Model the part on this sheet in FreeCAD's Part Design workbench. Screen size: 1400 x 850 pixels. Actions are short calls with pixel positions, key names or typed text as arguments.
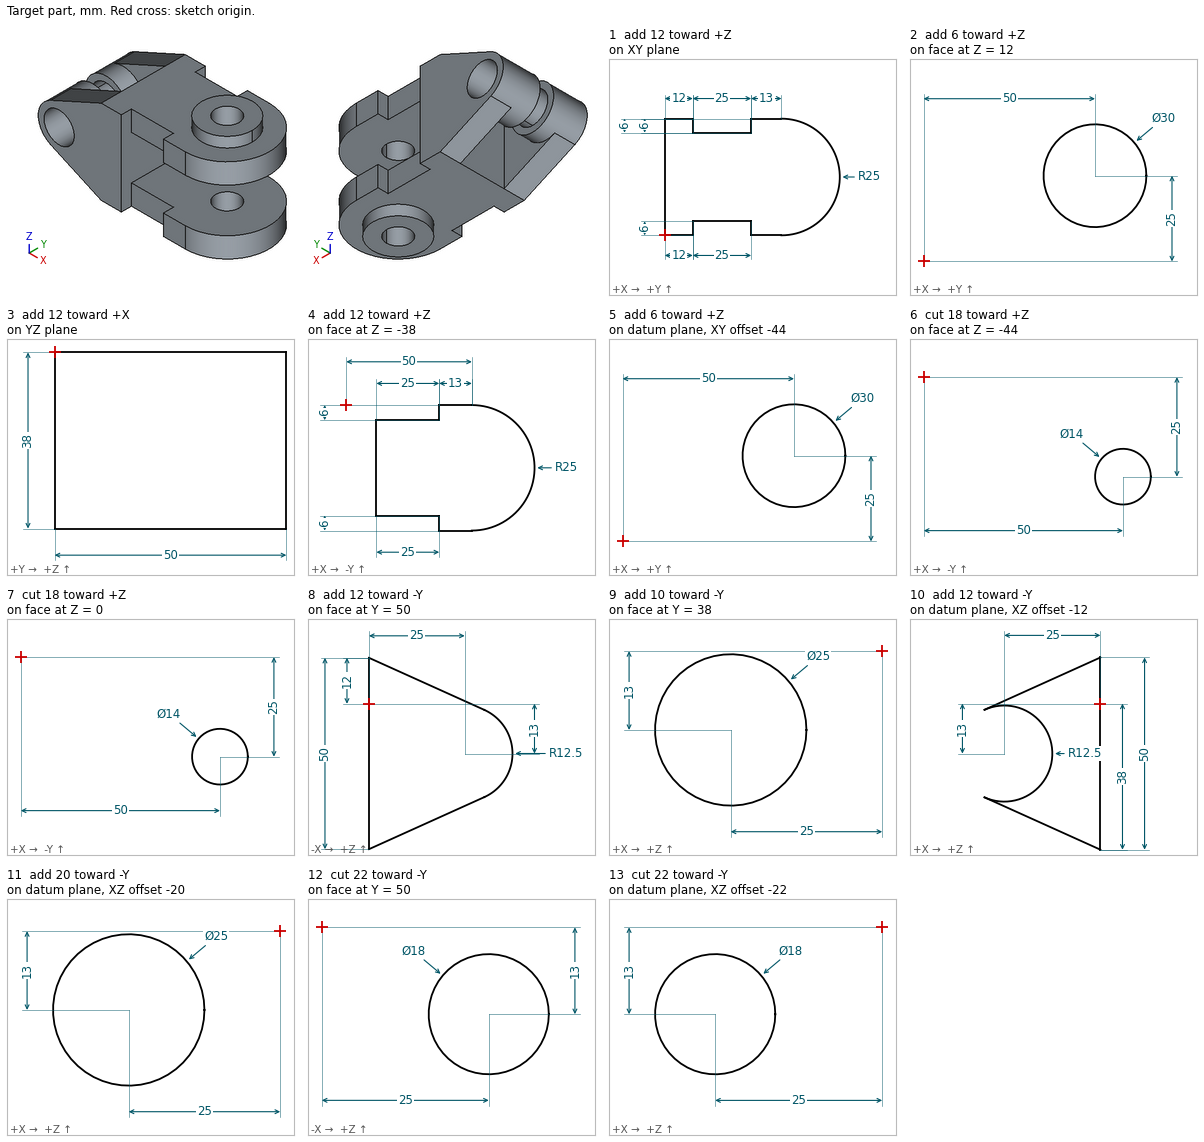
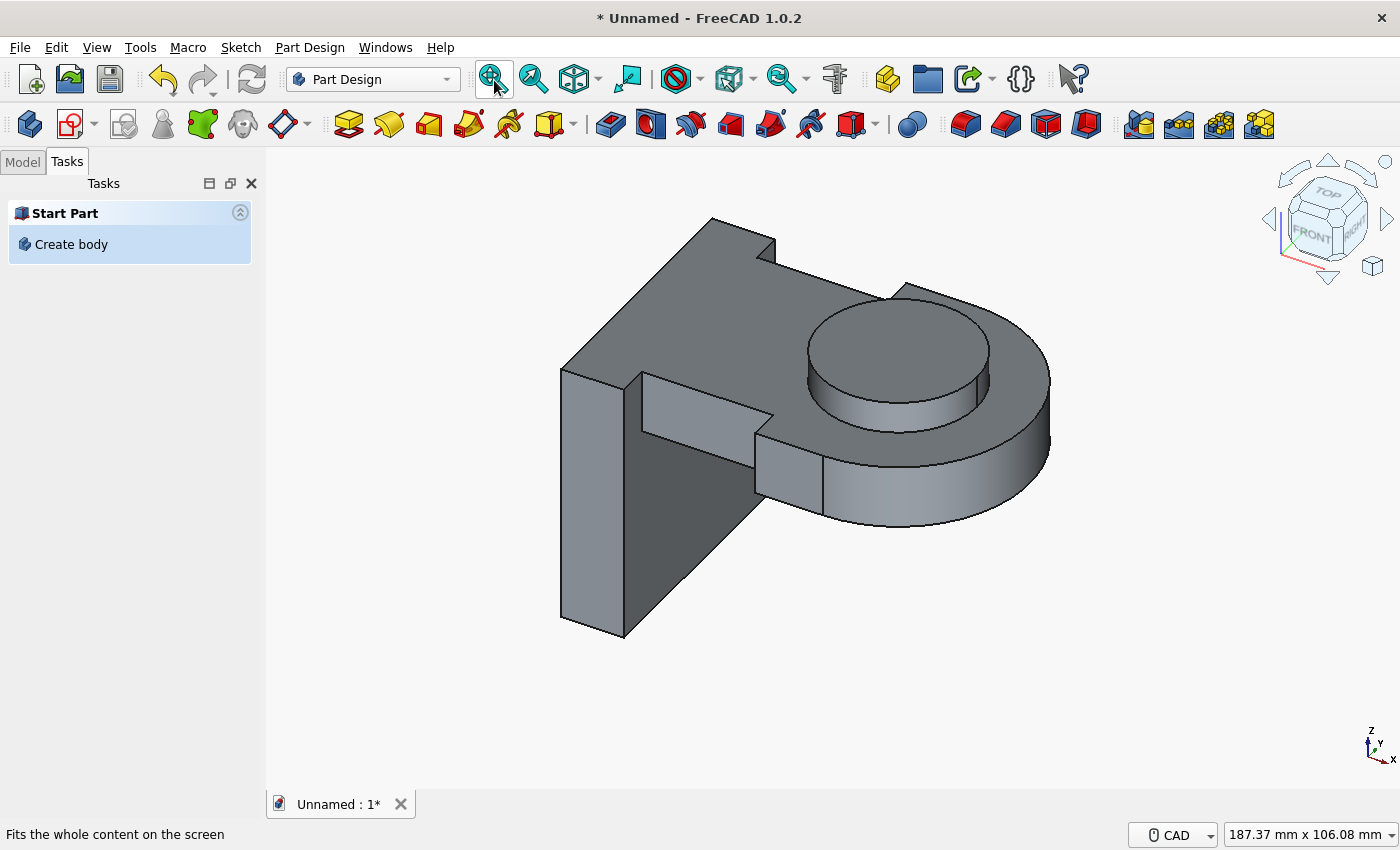
key(5)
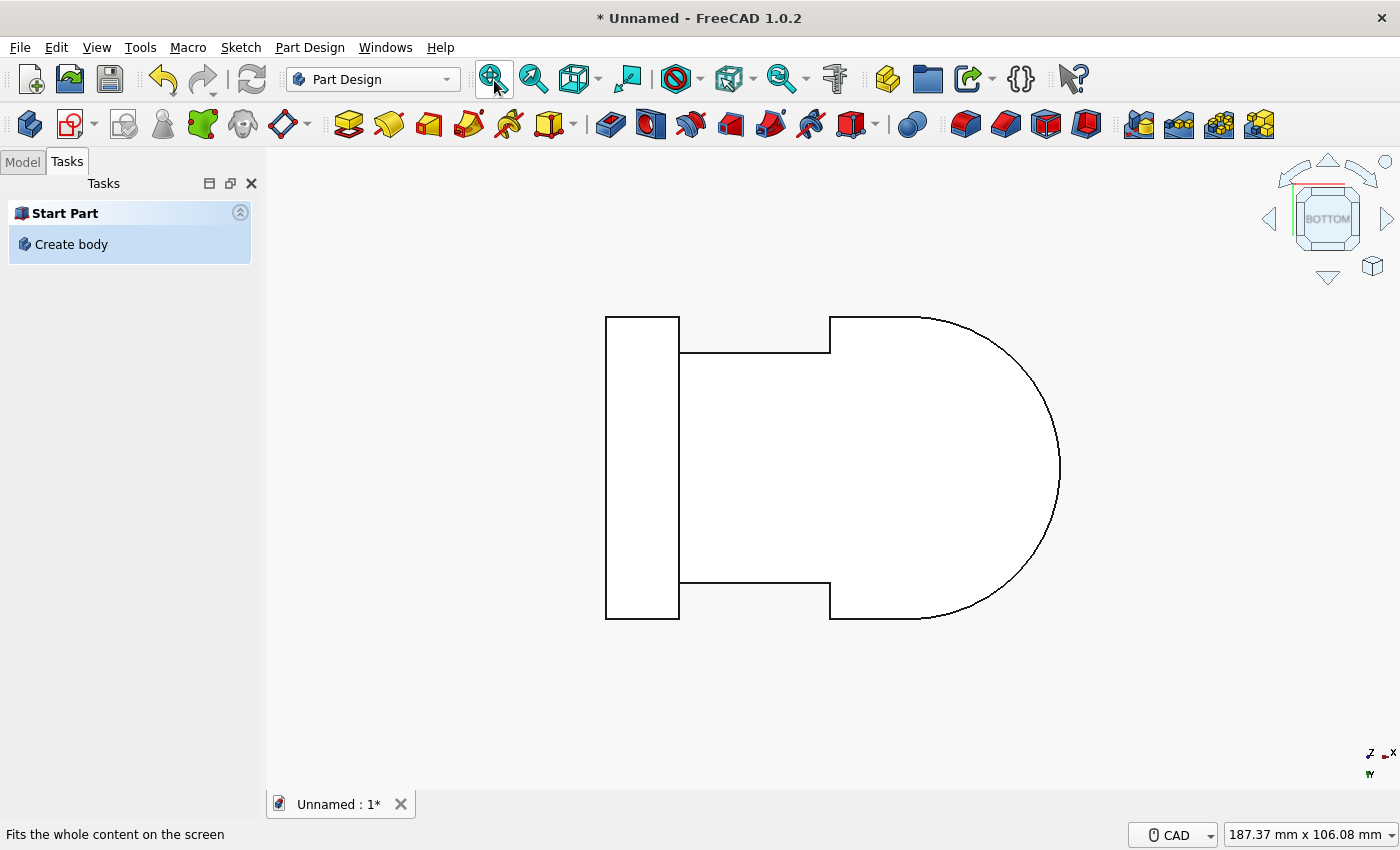
click(643, 553)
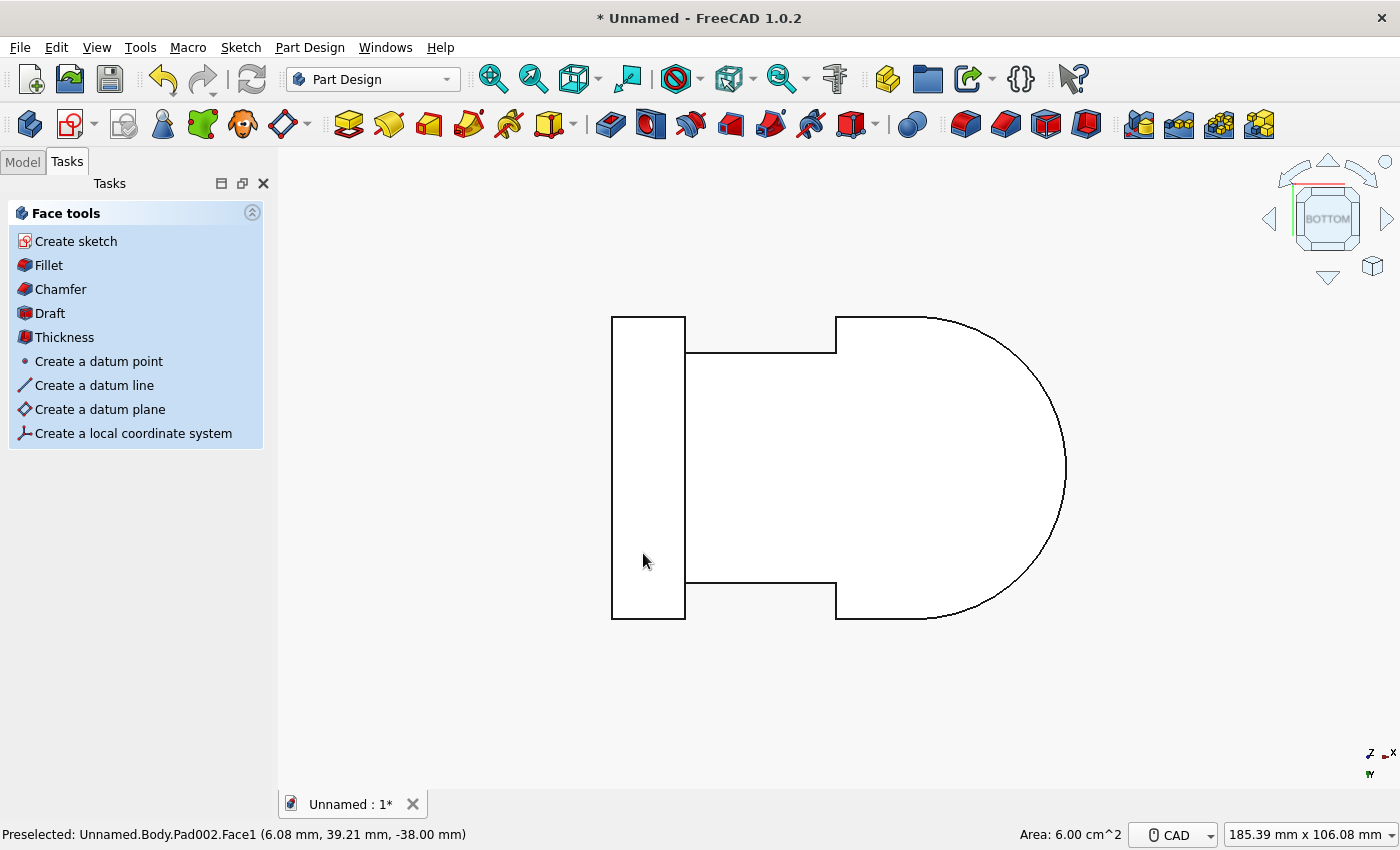
click(70, 124)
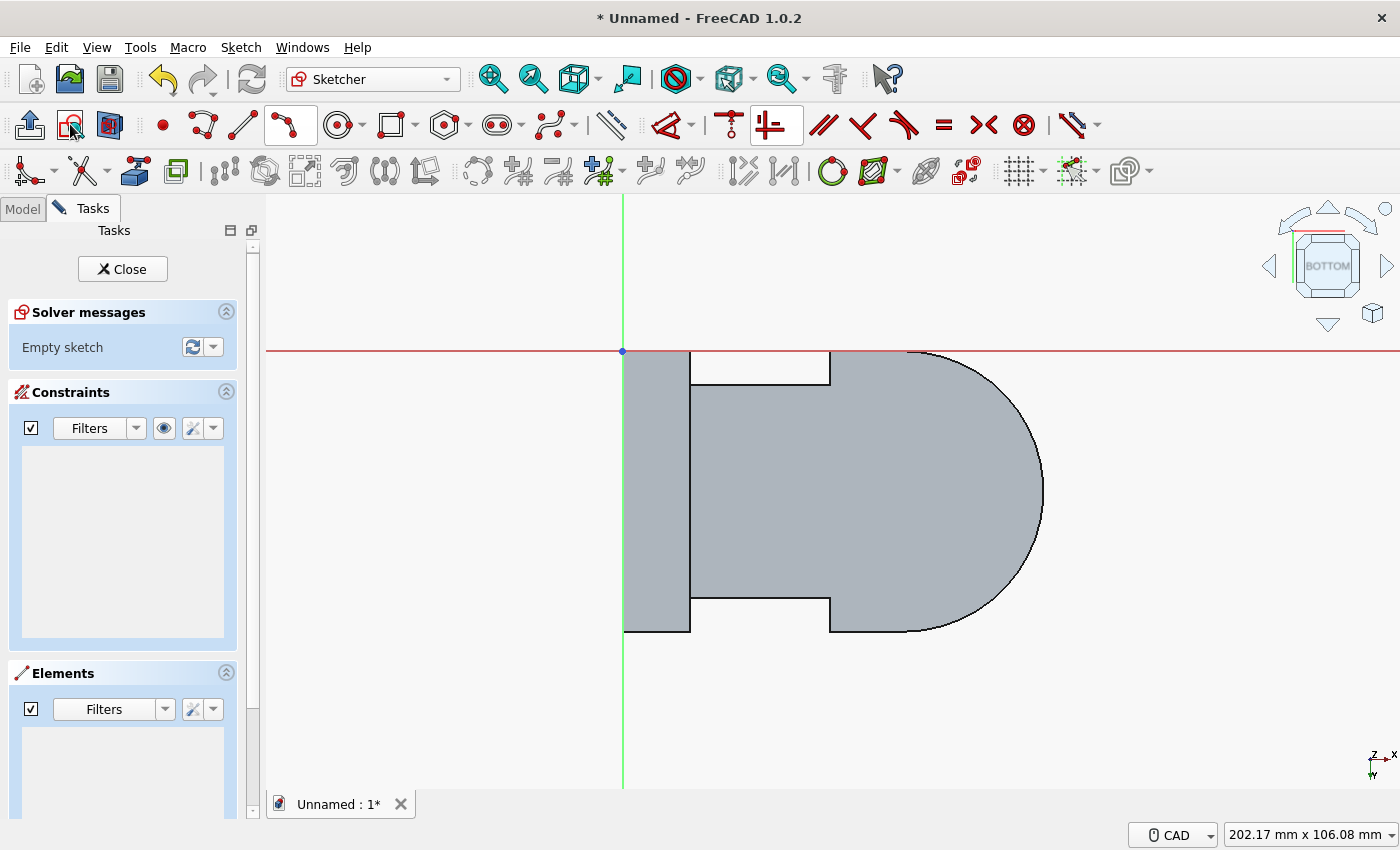
scroll(973, 491, up, 2)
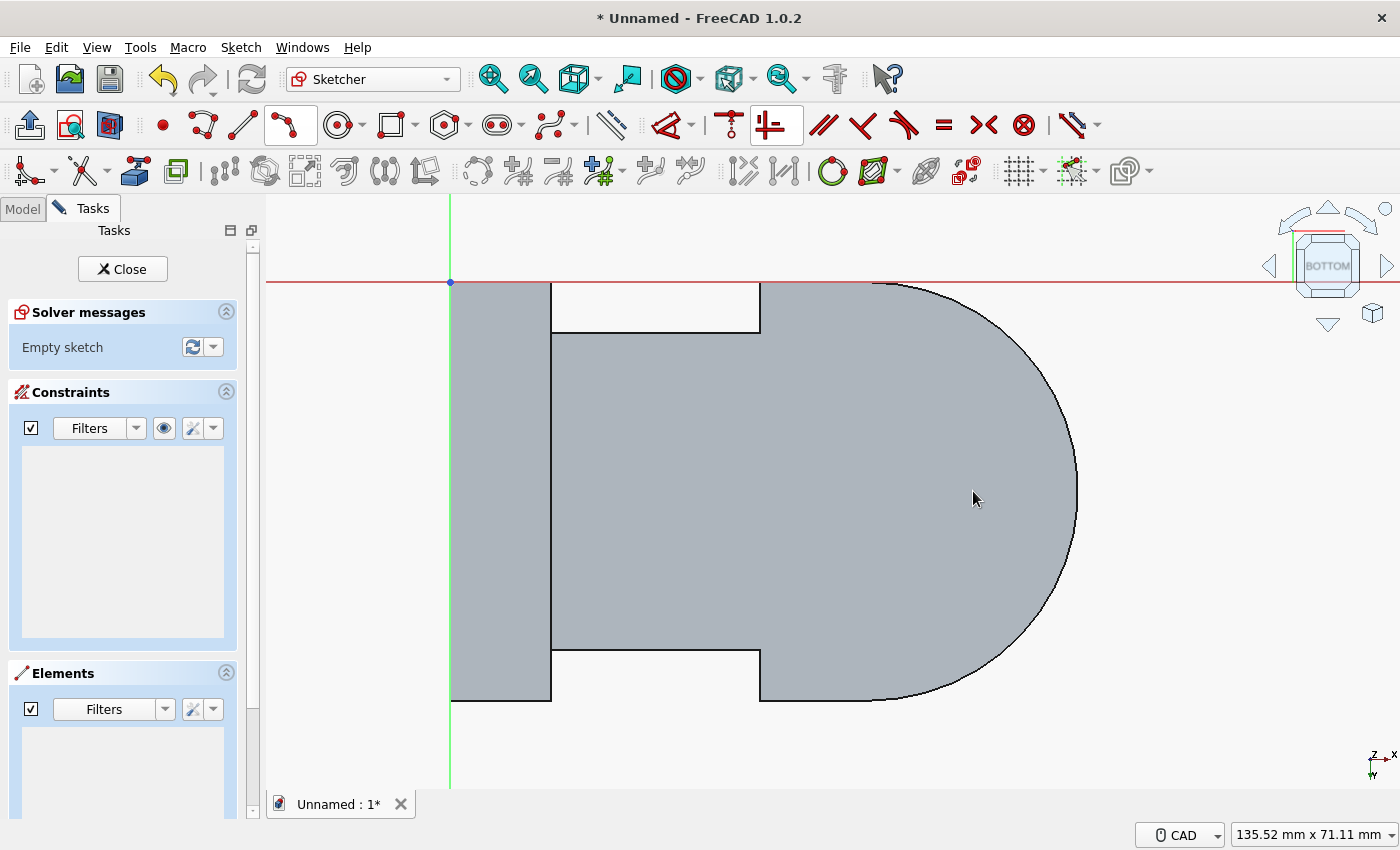
click(204, 126)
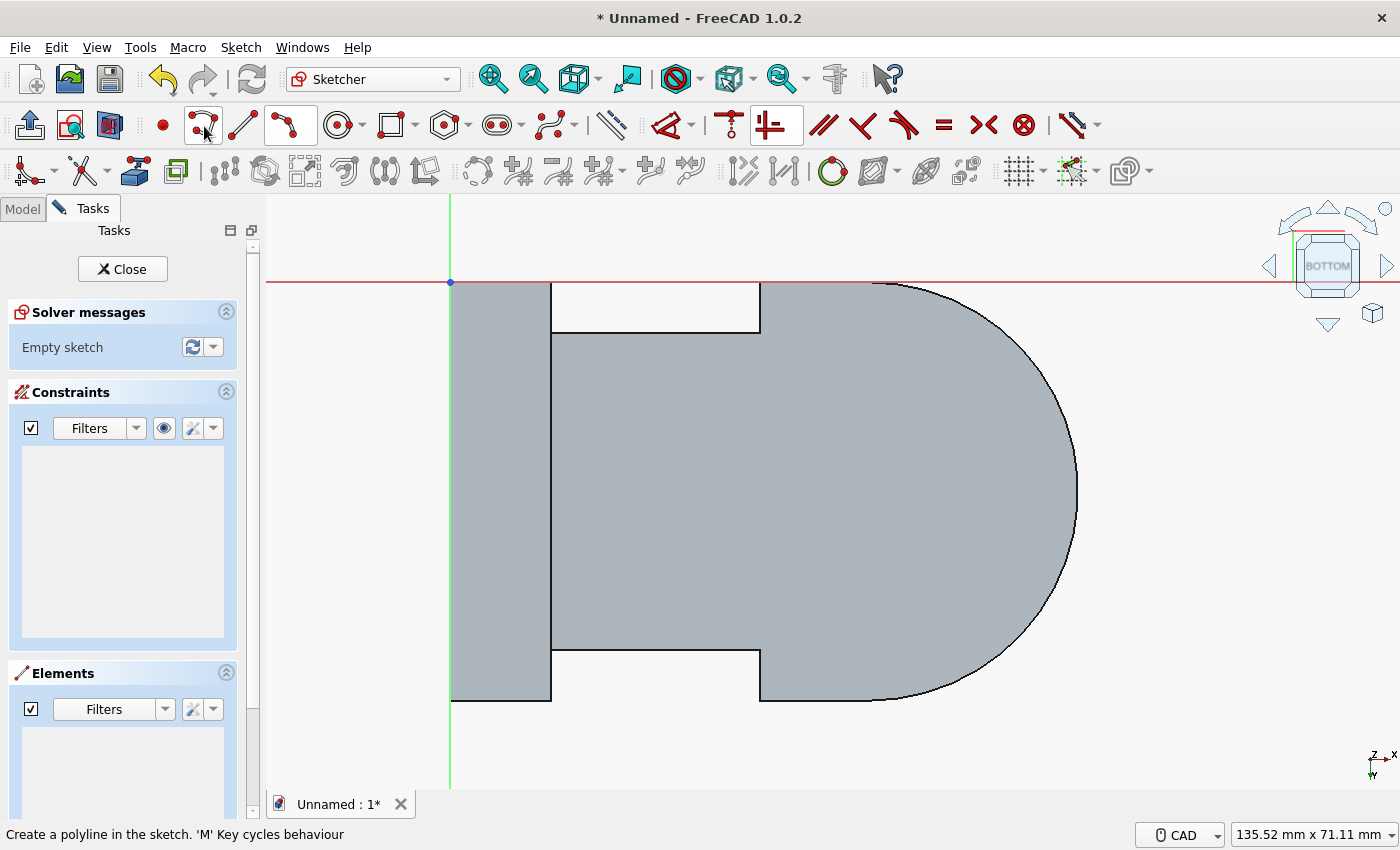
click(869, 282)
click(760, 291)
click(760, 333)
click(551, 333)
click(551, 650)
click(760, 650)
click(760, 701)
click(869, 701)
right_click(869, 701)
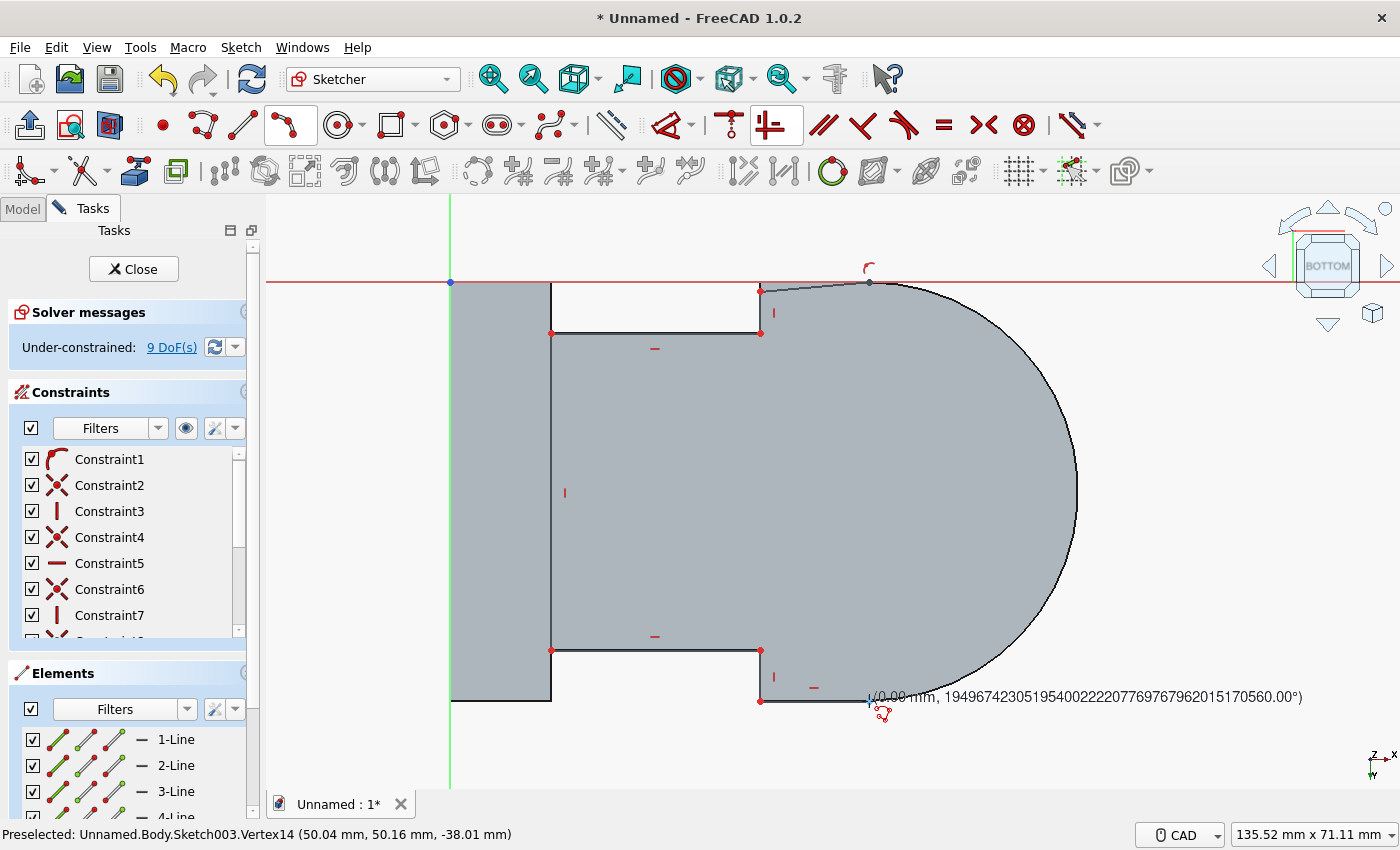
key(g)
key(3)
key(a)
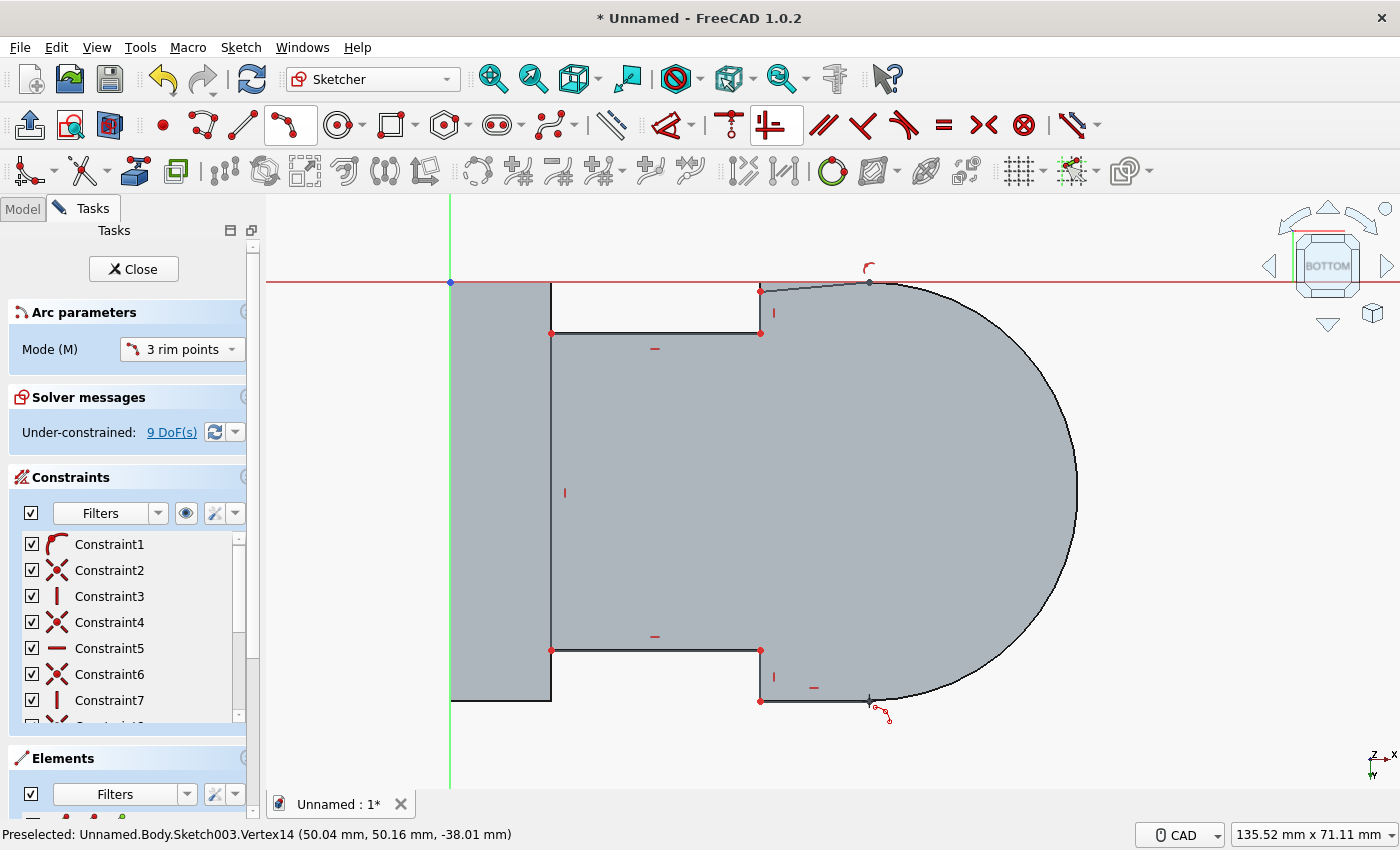
click(869, 702)
click(869, 282)
click(1078, 492)
key(Escape)